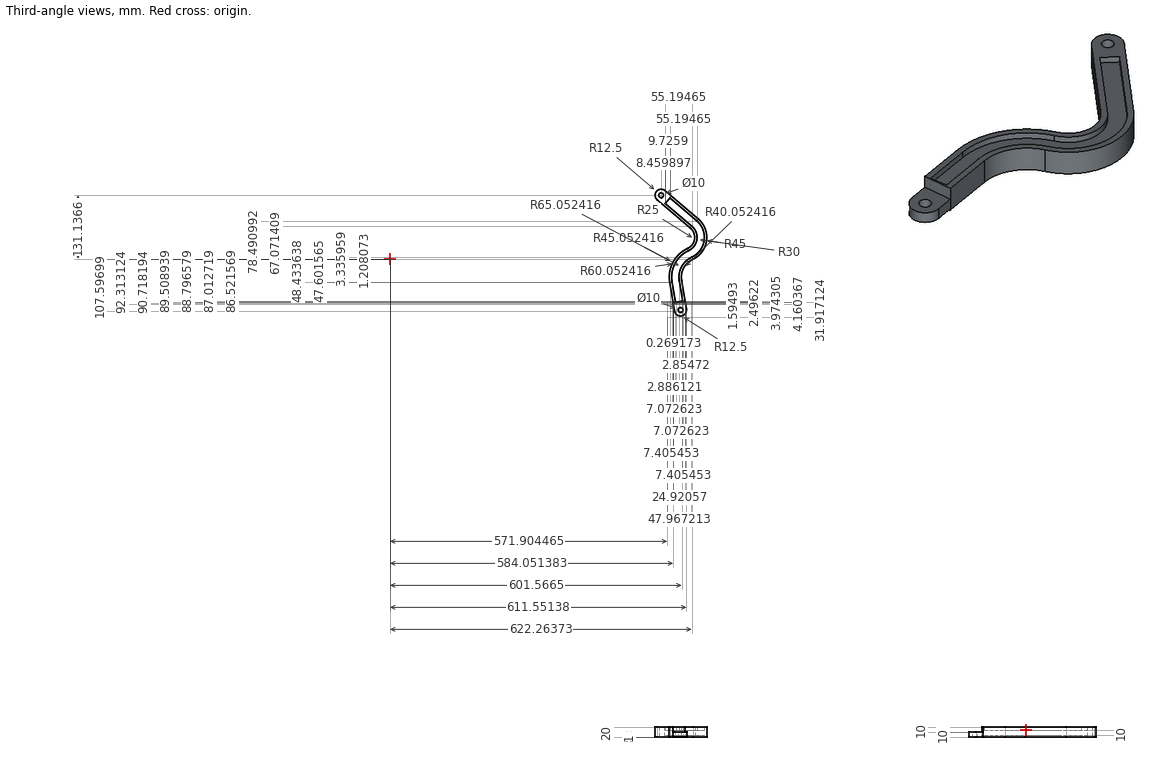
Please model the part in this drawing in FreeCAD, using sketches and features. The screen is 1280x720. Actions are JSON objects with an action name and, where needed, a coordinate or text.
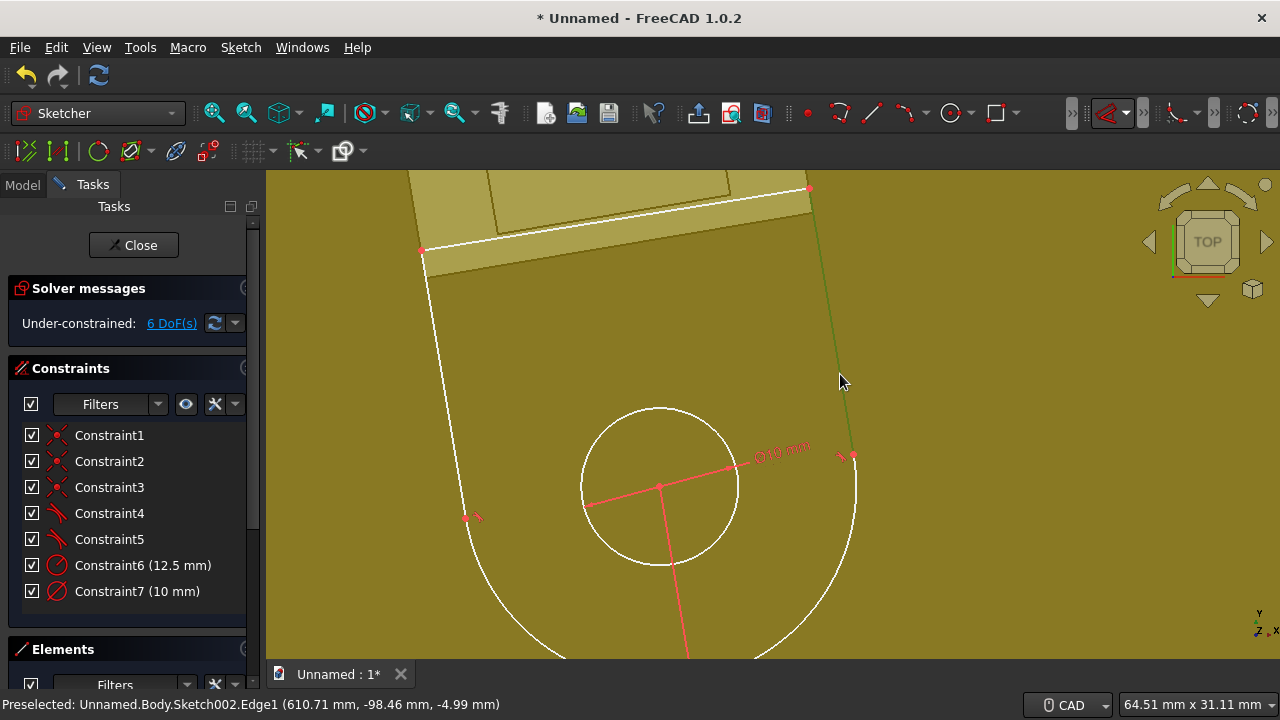
{"action": "key", "text": "l"}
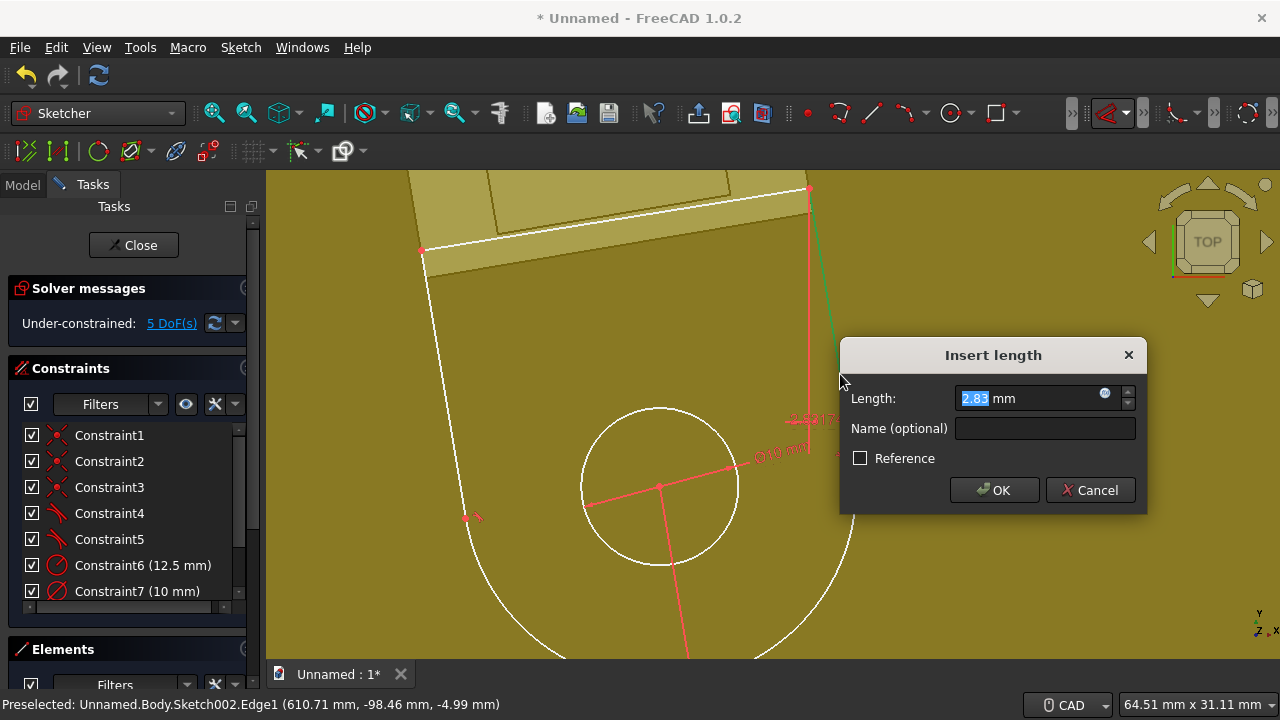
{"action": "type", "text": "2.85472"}
{"action": "key", "text": "Return"}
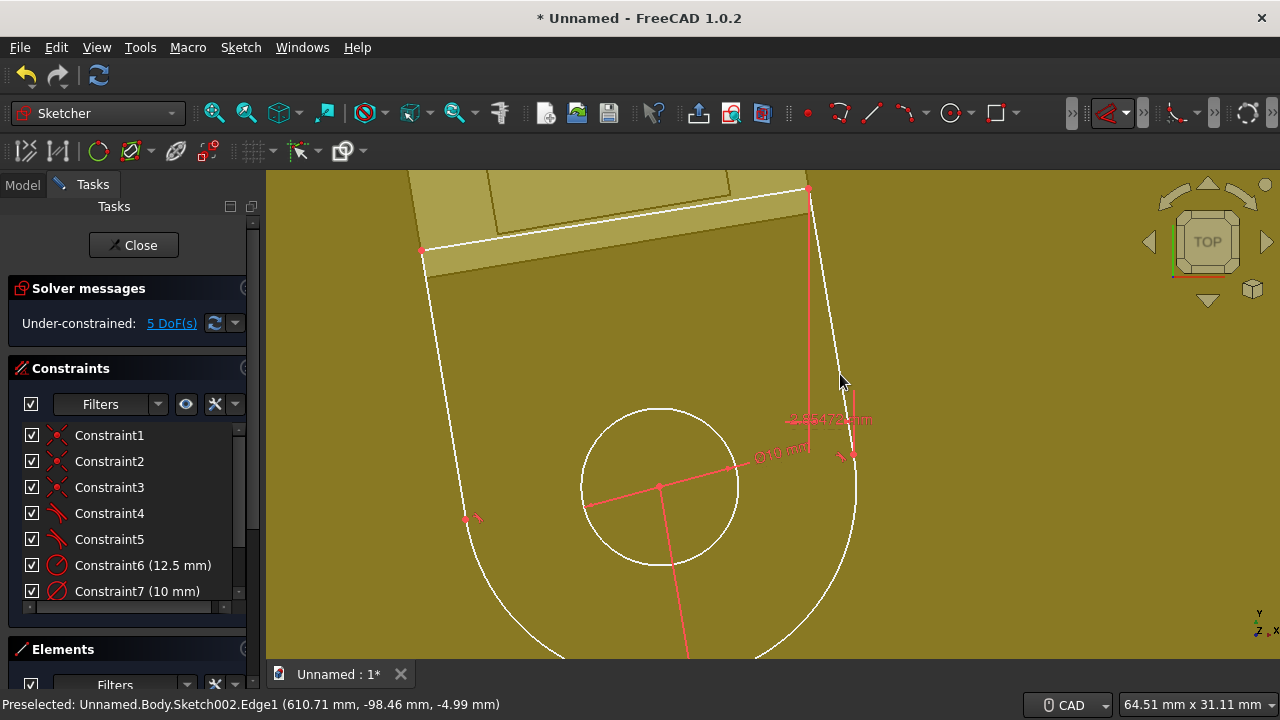
{"action": "left_click", "coordinate": [692, 207]}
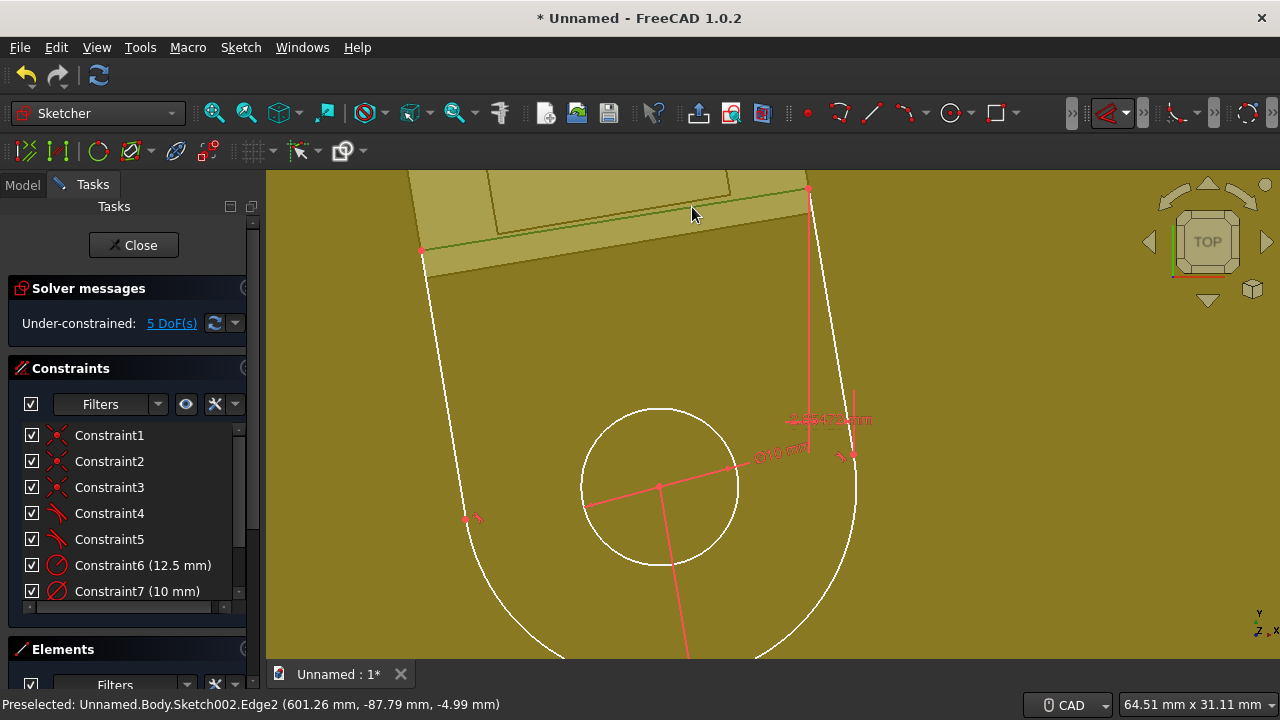
{"action": "key", "text": "i"}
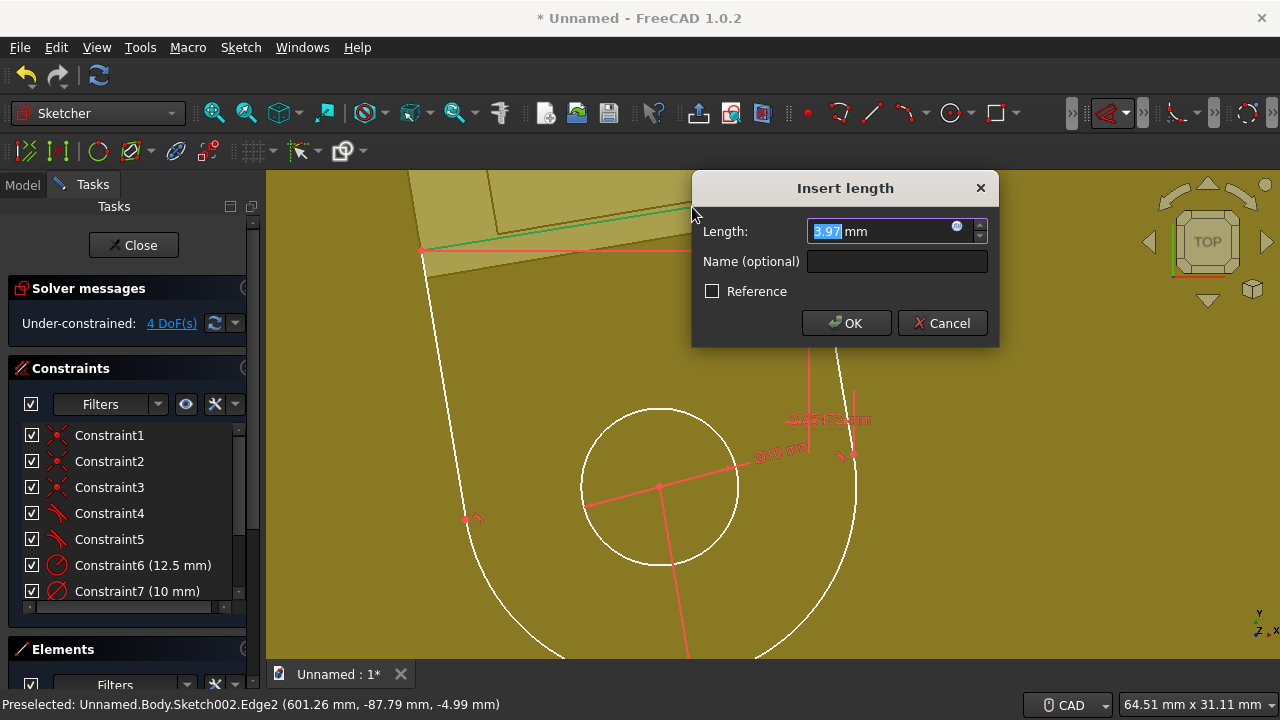
{"action": "type", "text": "3.974305"}
{"action": "key", "text": "Return"}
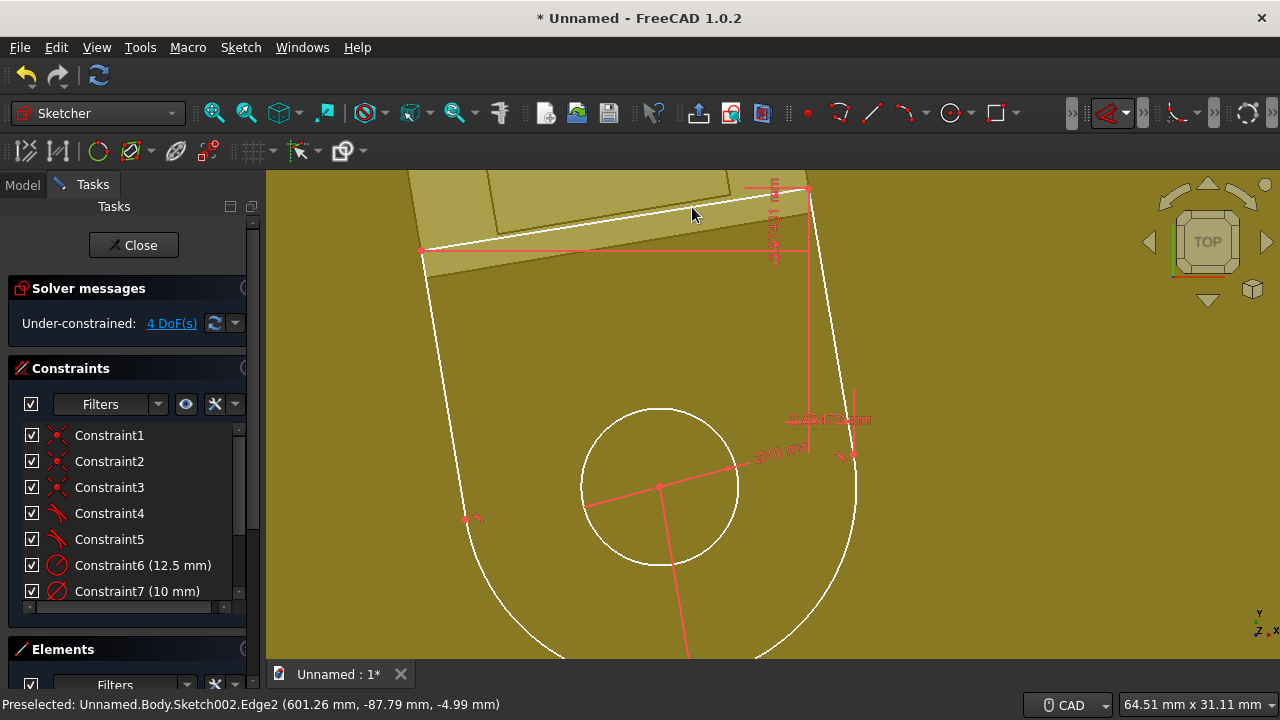
{"action": "left_click", "coordinate": [435, 331]}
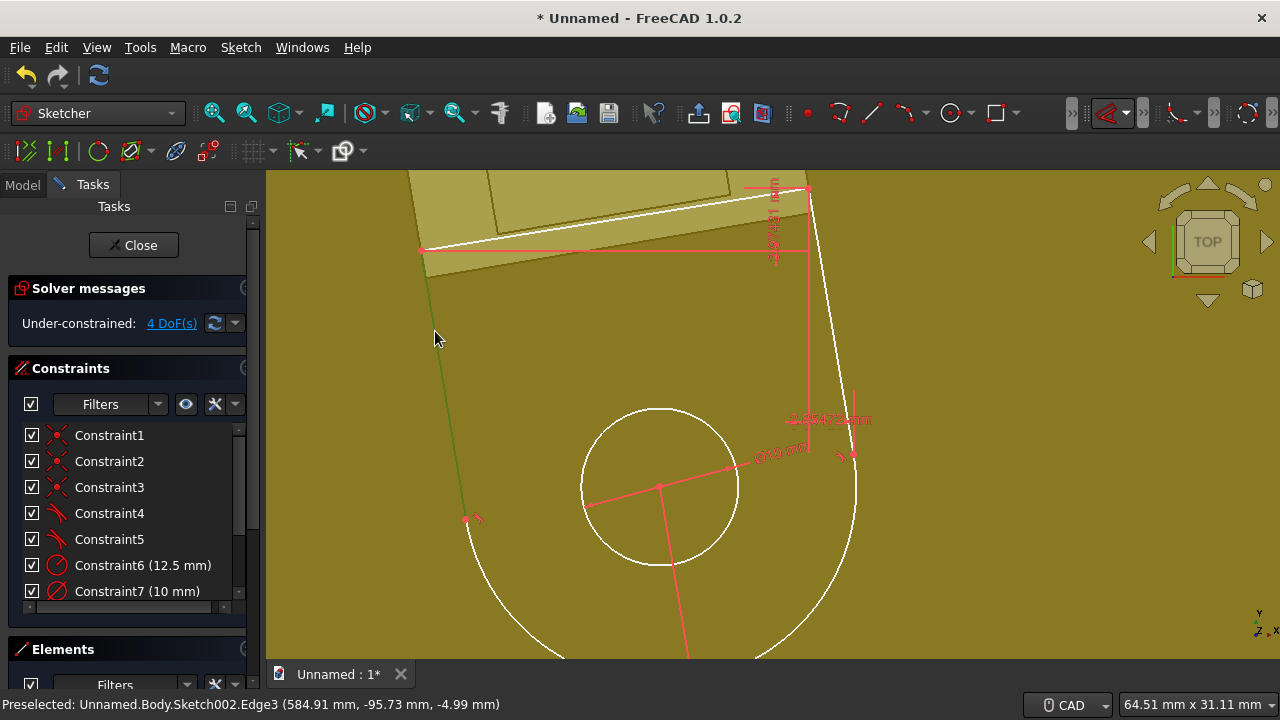
{"action": "left_click", "coordinate": [1128, 114]}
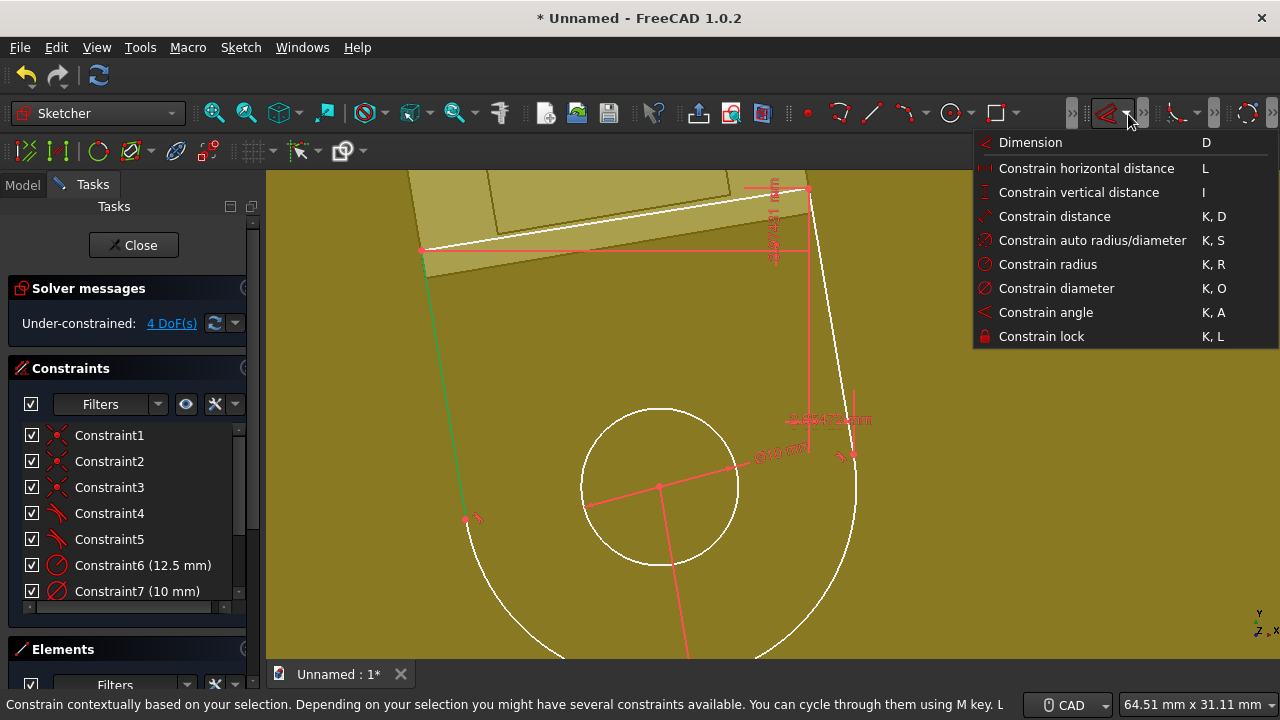
{"action": "left_click", "coordinate": [1126, 168]}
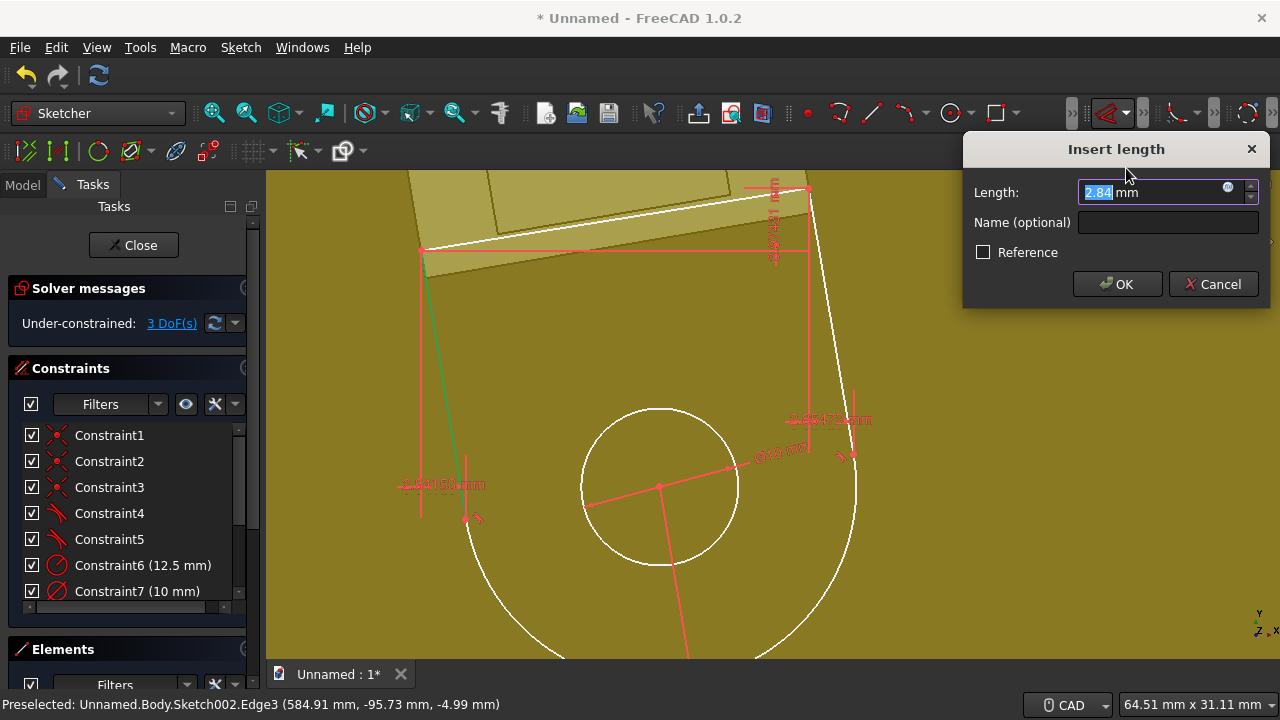
{"action": "type", "text": "2.886121"}
{"action": "key", "text": "Return"}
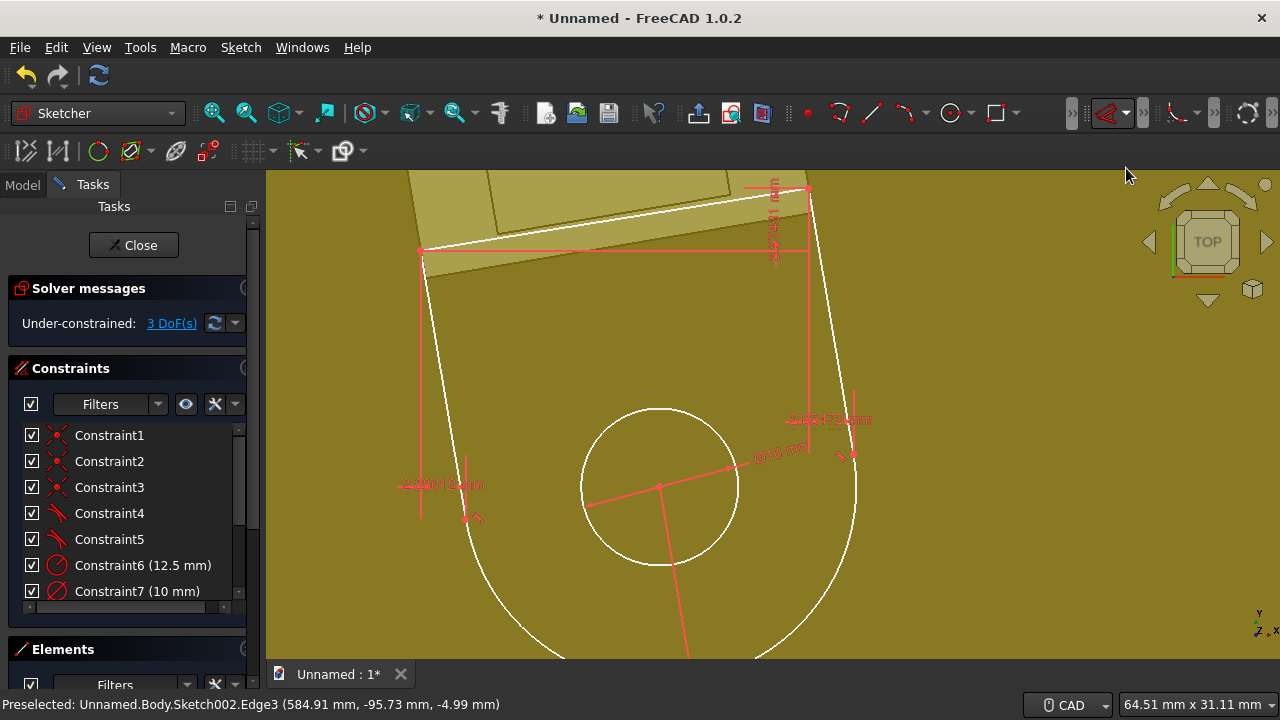
{"action": "left_click", "coordinate": [854, 454]}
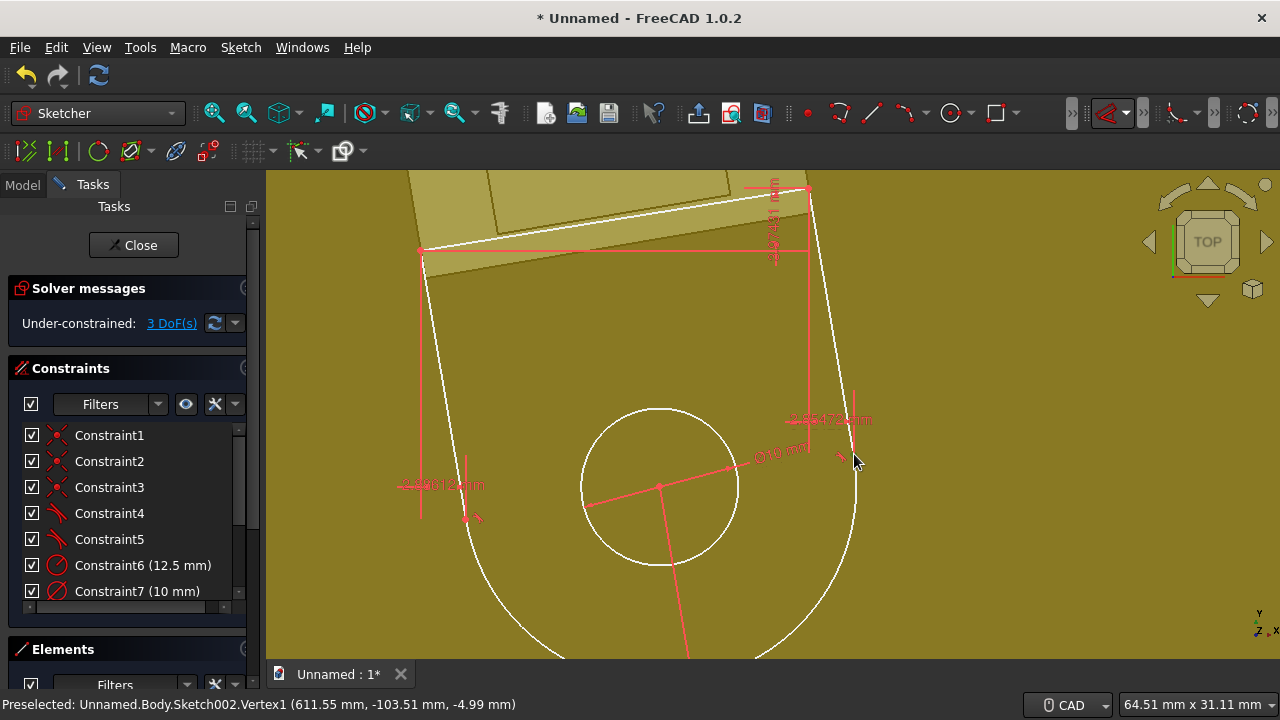
{"action": "left_click", "coordinate": [1128, 114]}